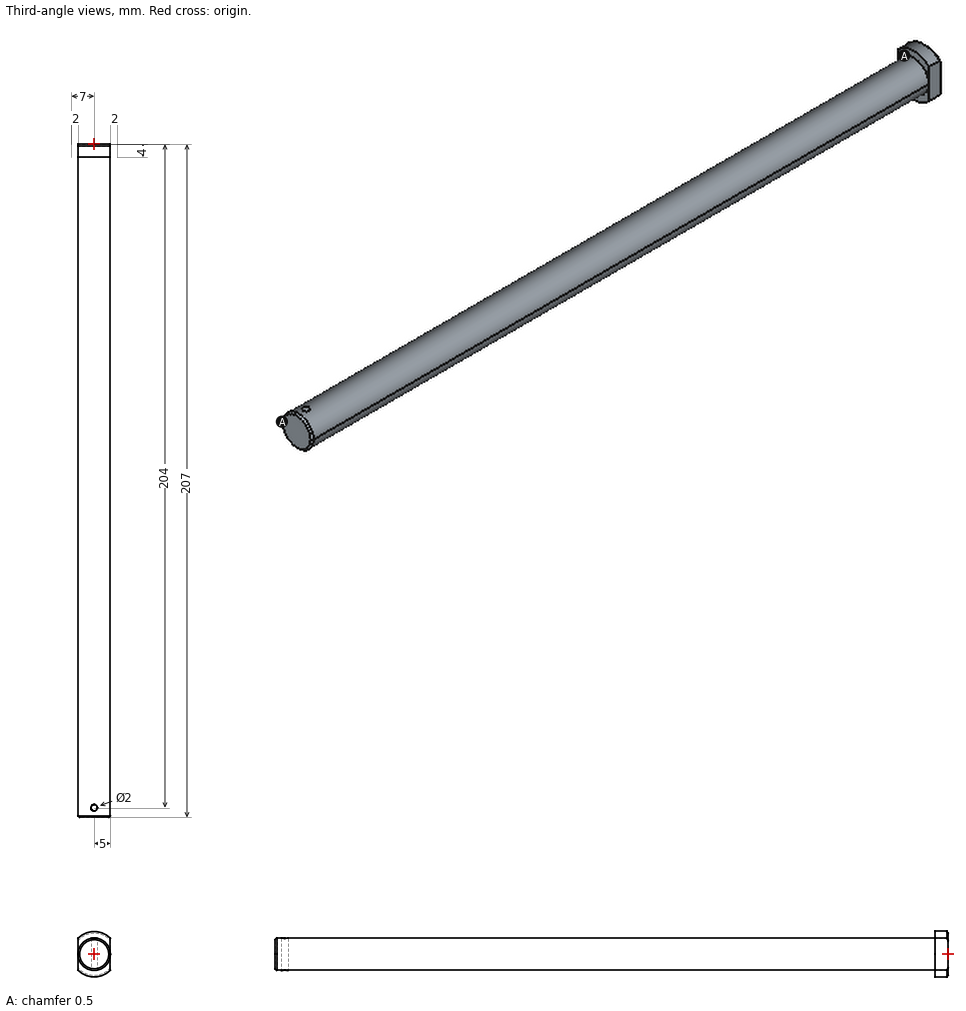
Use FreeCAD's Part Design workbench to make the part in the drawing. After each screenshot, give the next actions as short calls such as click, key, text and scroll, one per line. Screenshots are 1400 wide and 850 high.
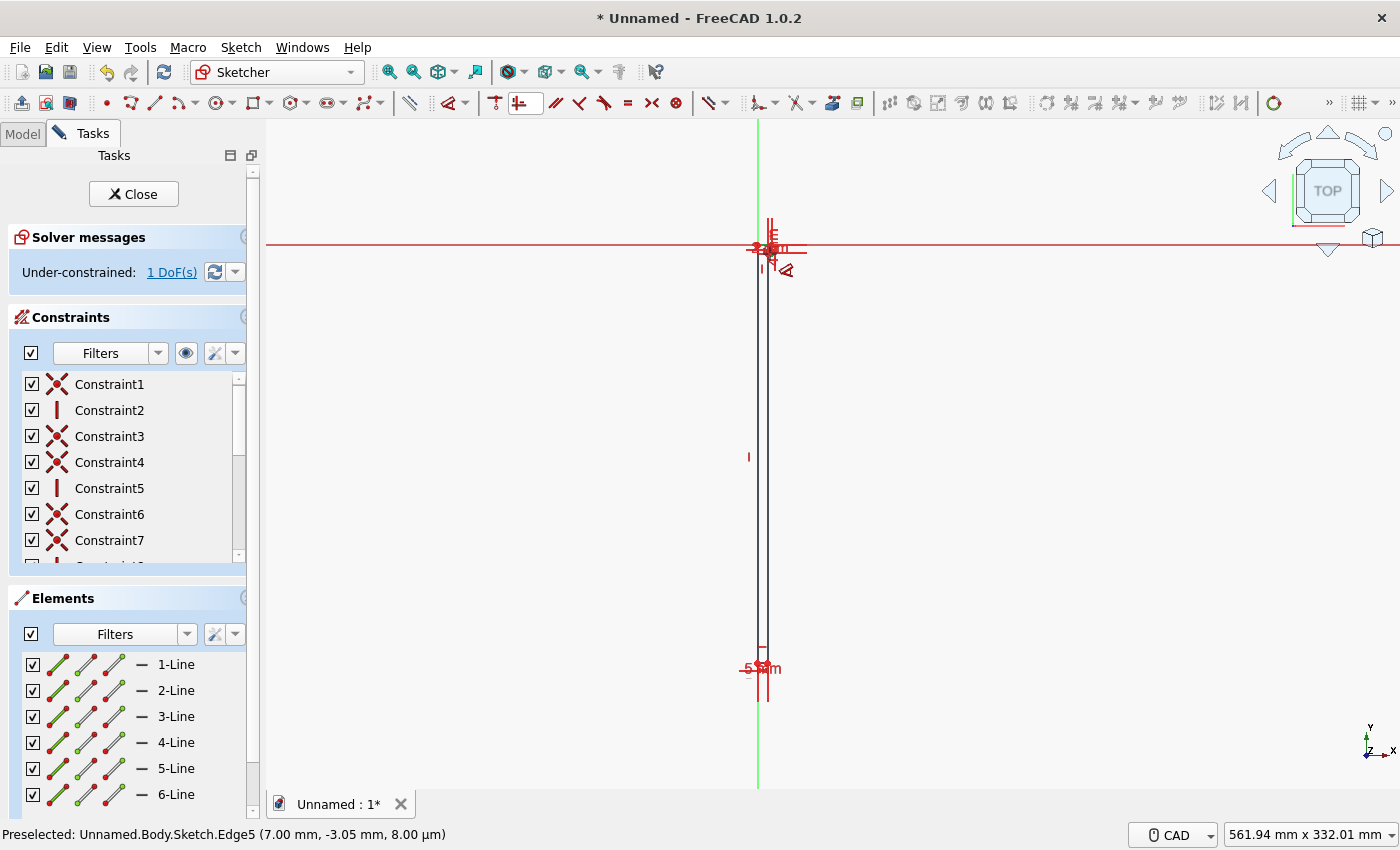
scroll(758, 371, up, 2)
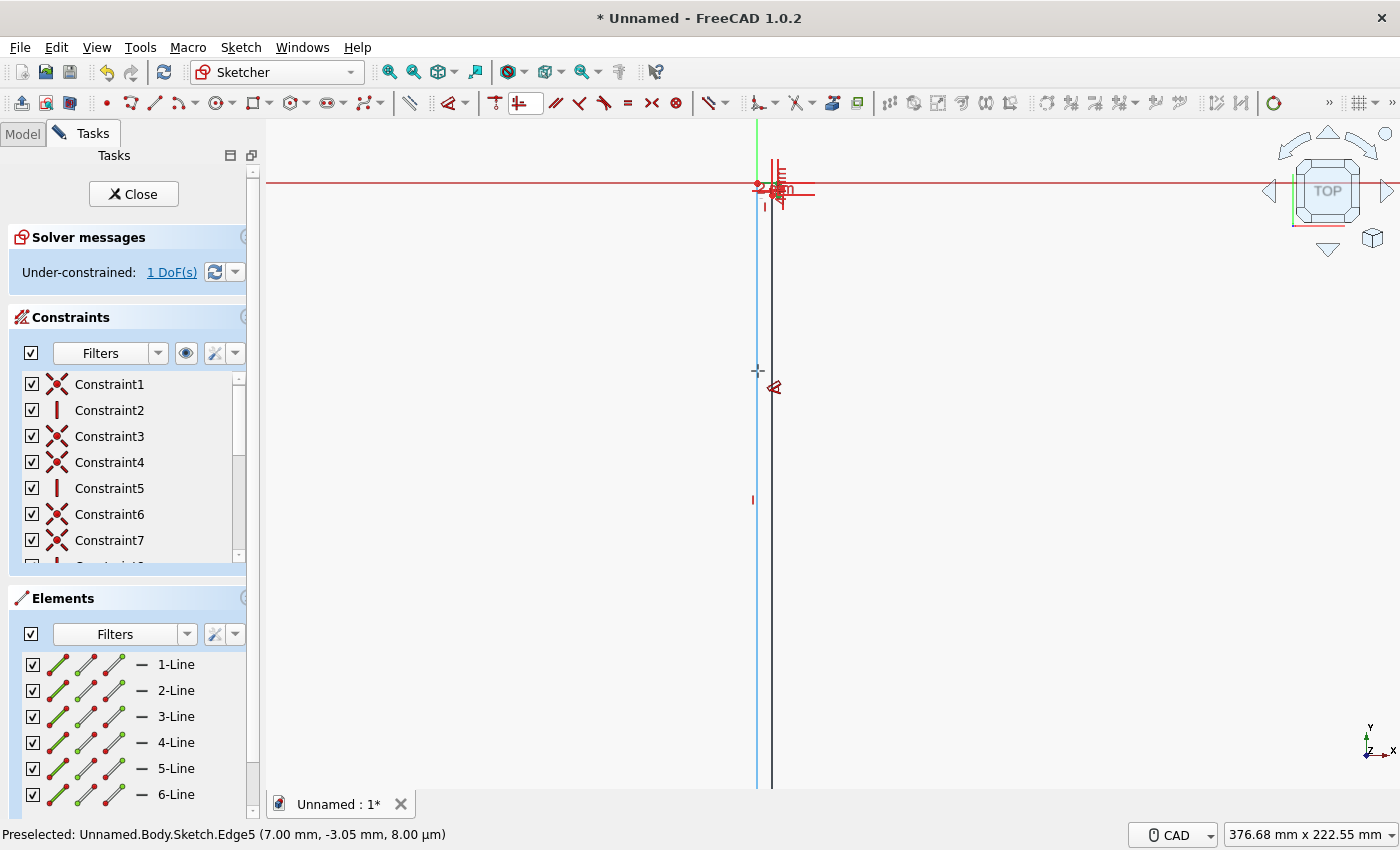
click(757, 370)
click(723, 472)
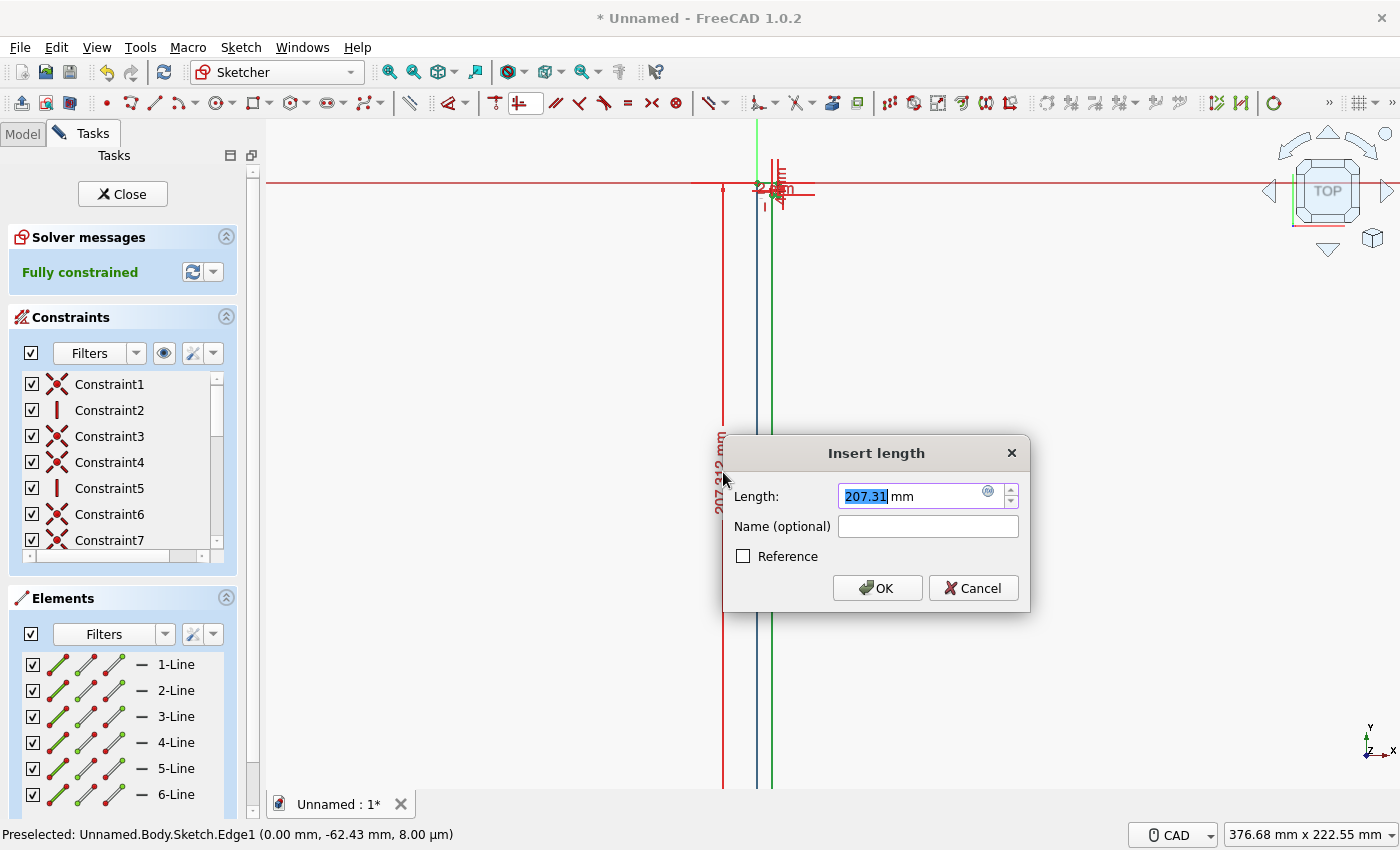
text(207)
key(Return)
key(Escape)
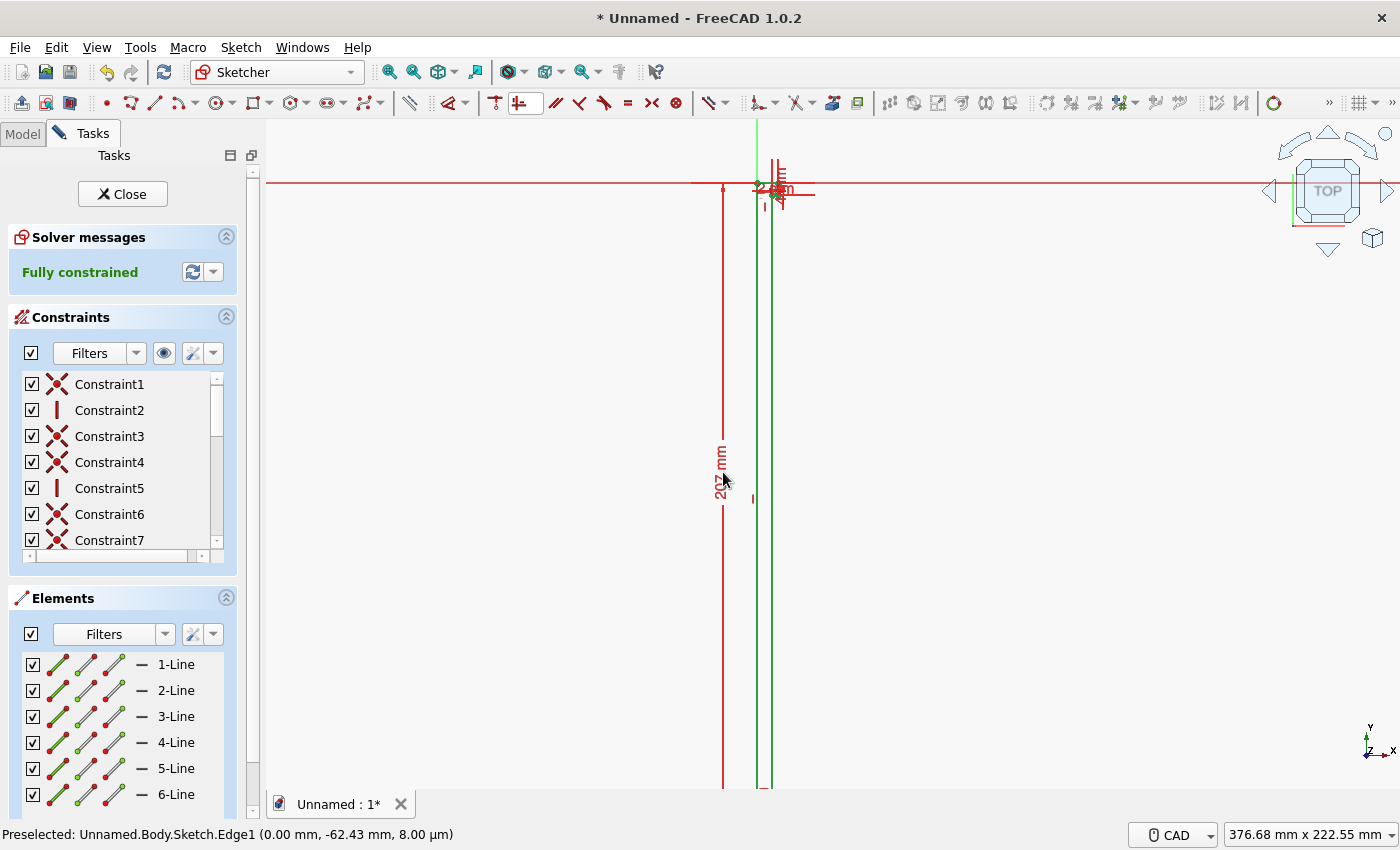
click(123, 194)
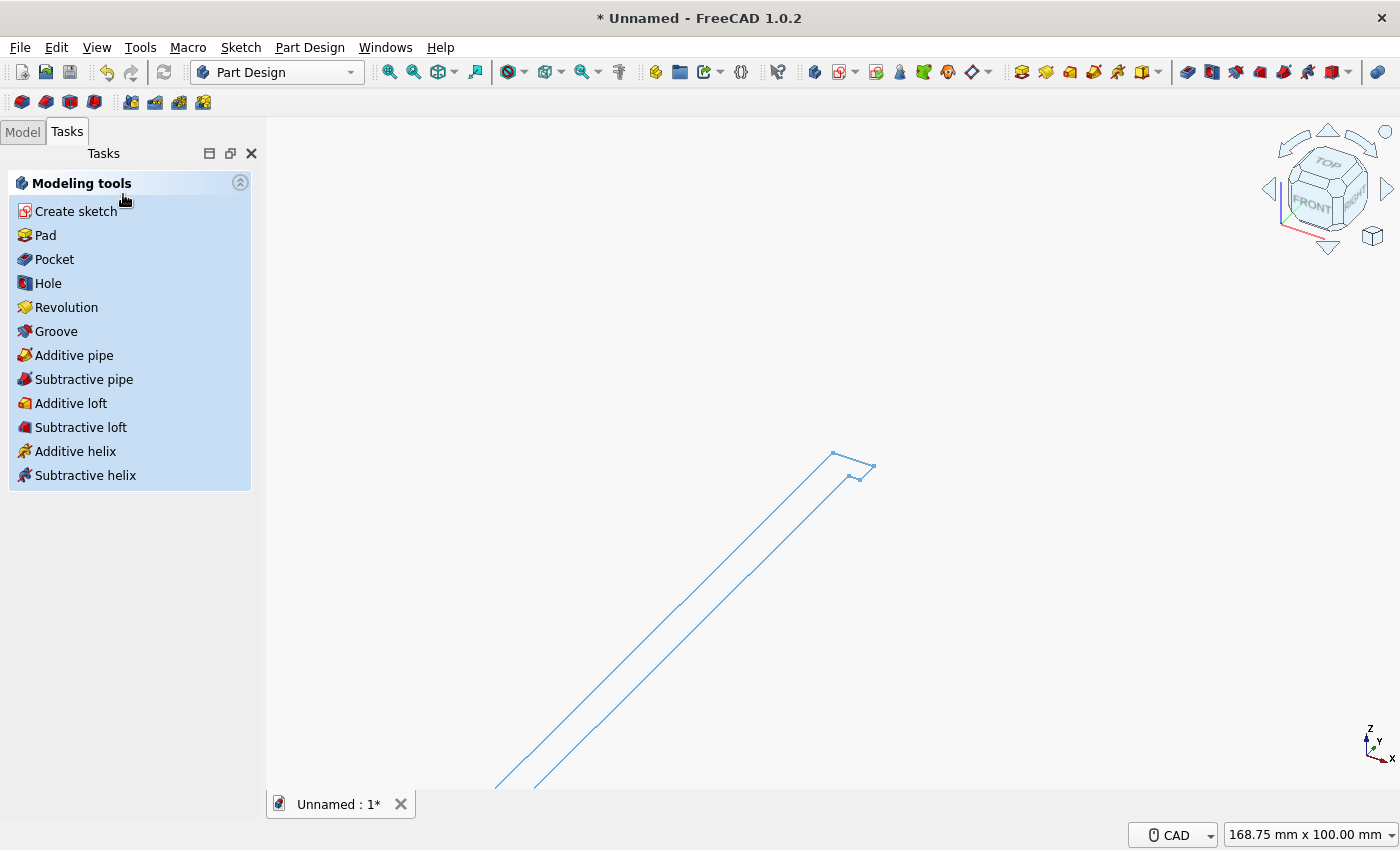
click(1046, 72)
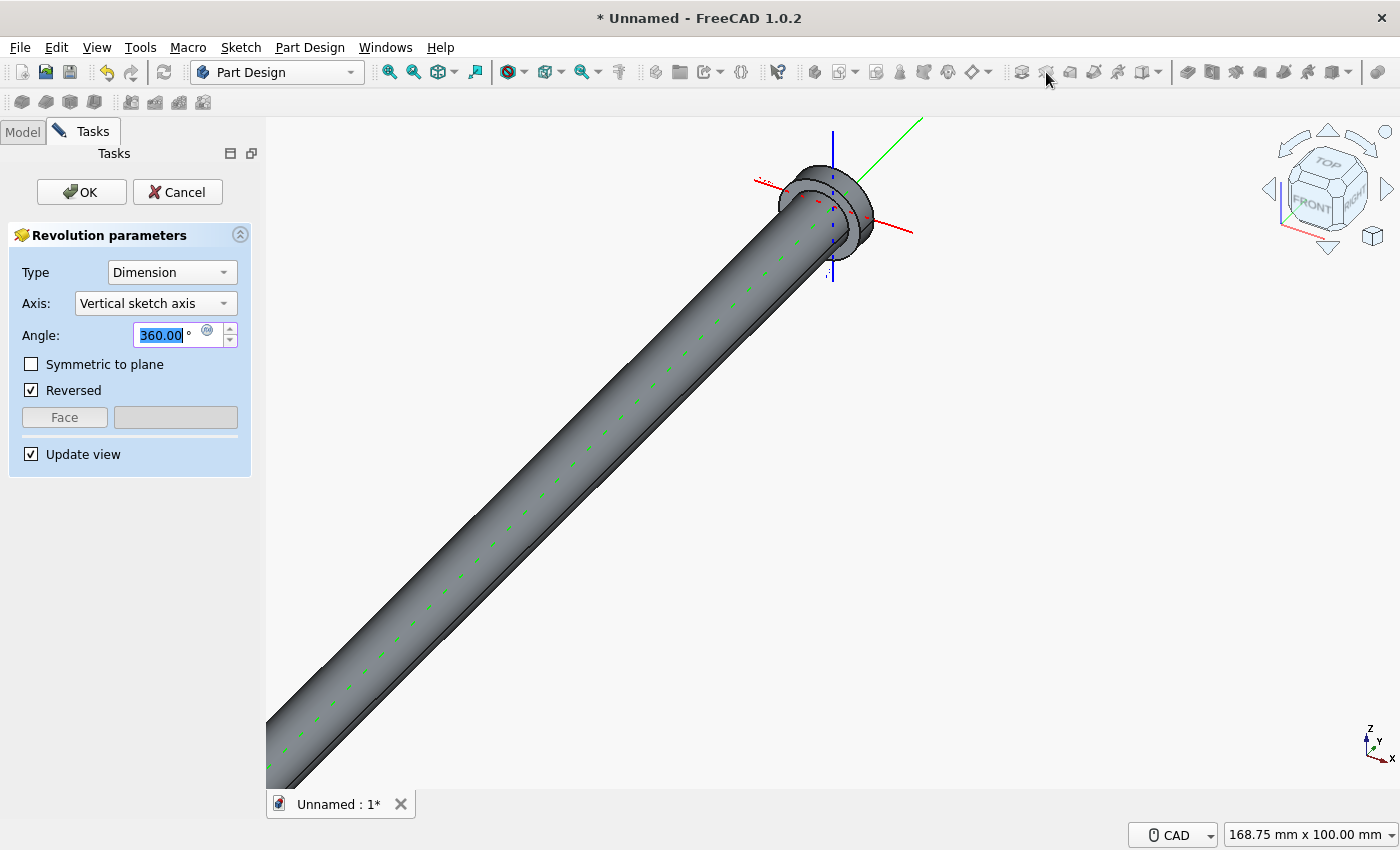
click(82, 192)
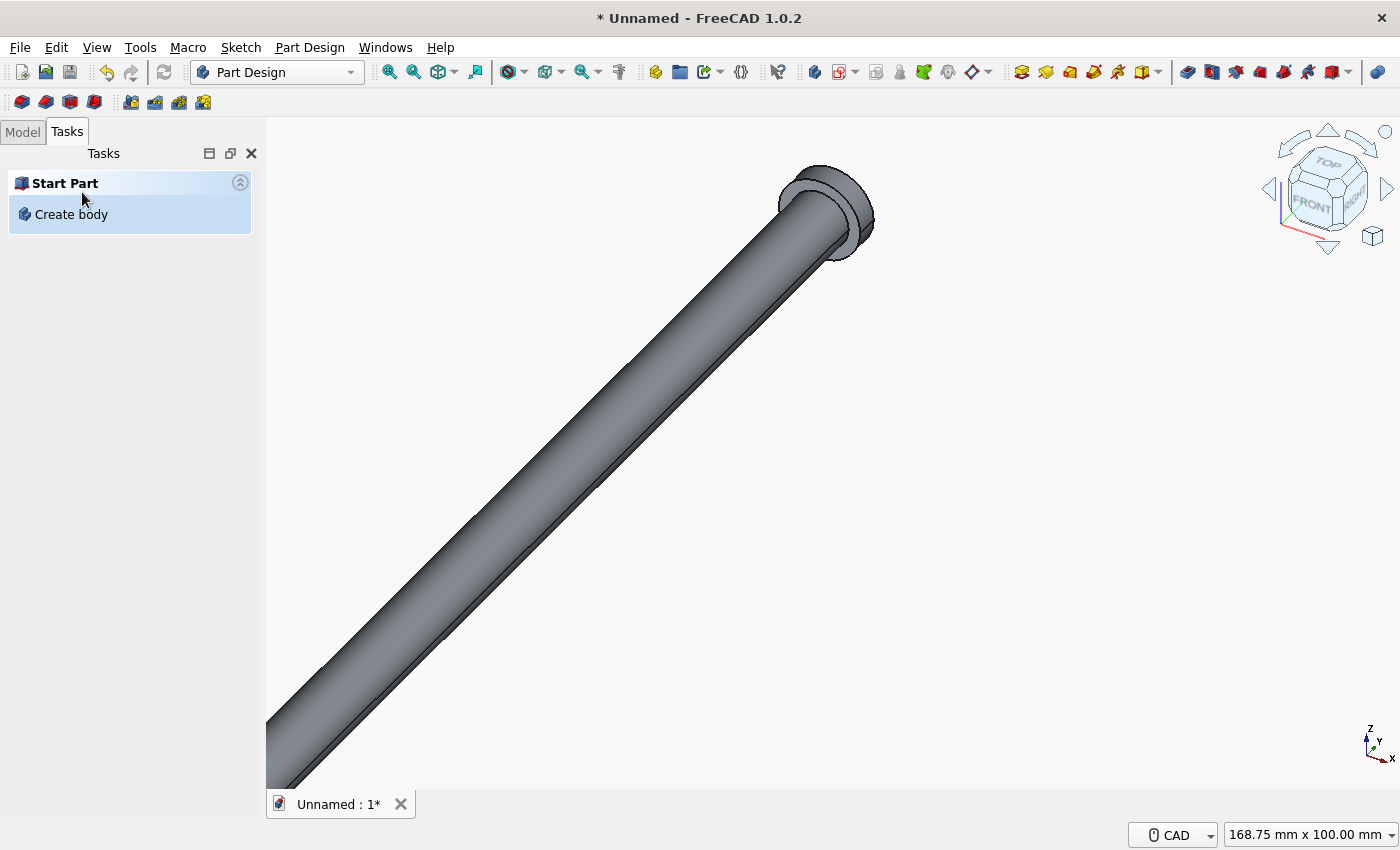
click(390, 72)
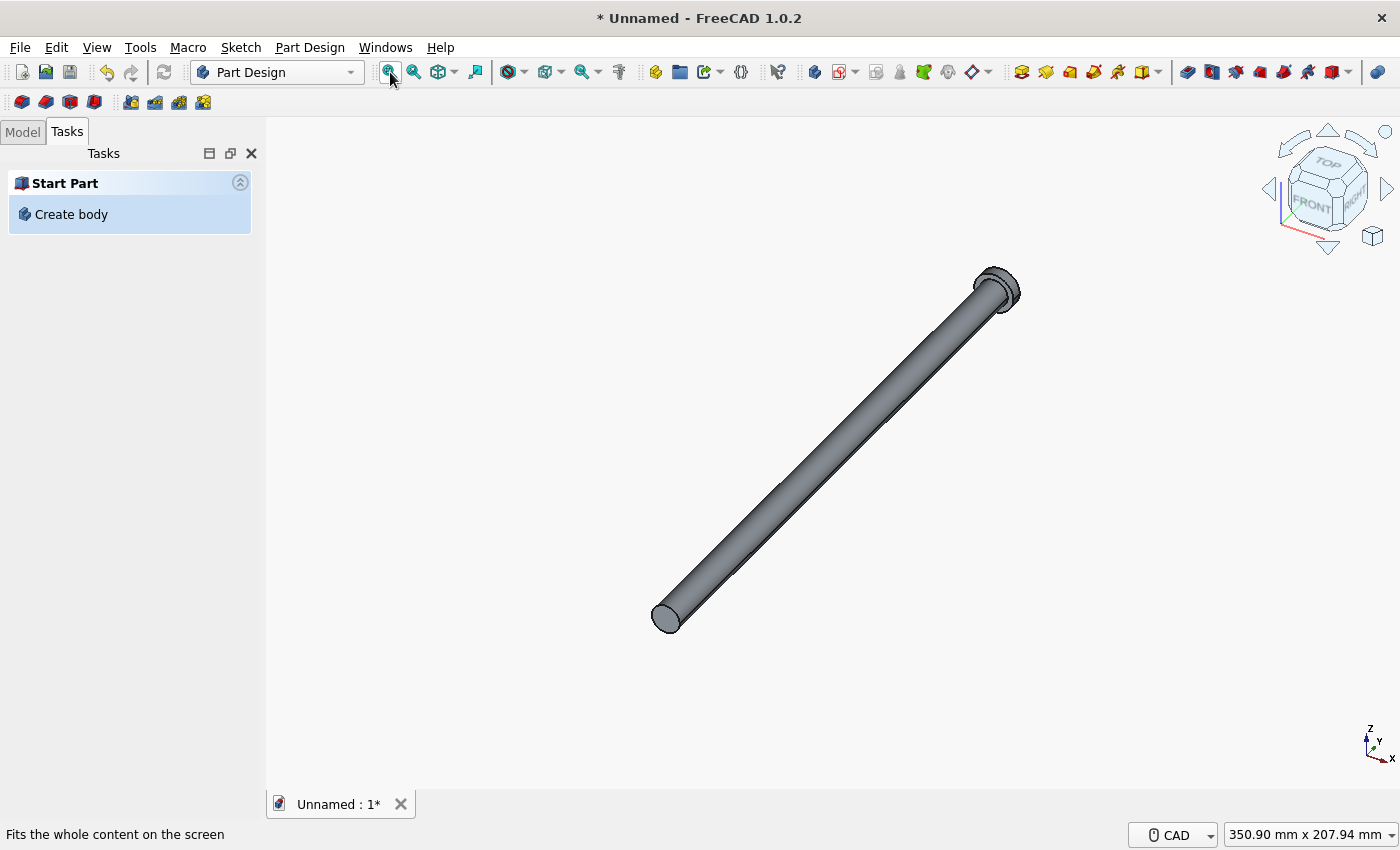
click(652, 614)